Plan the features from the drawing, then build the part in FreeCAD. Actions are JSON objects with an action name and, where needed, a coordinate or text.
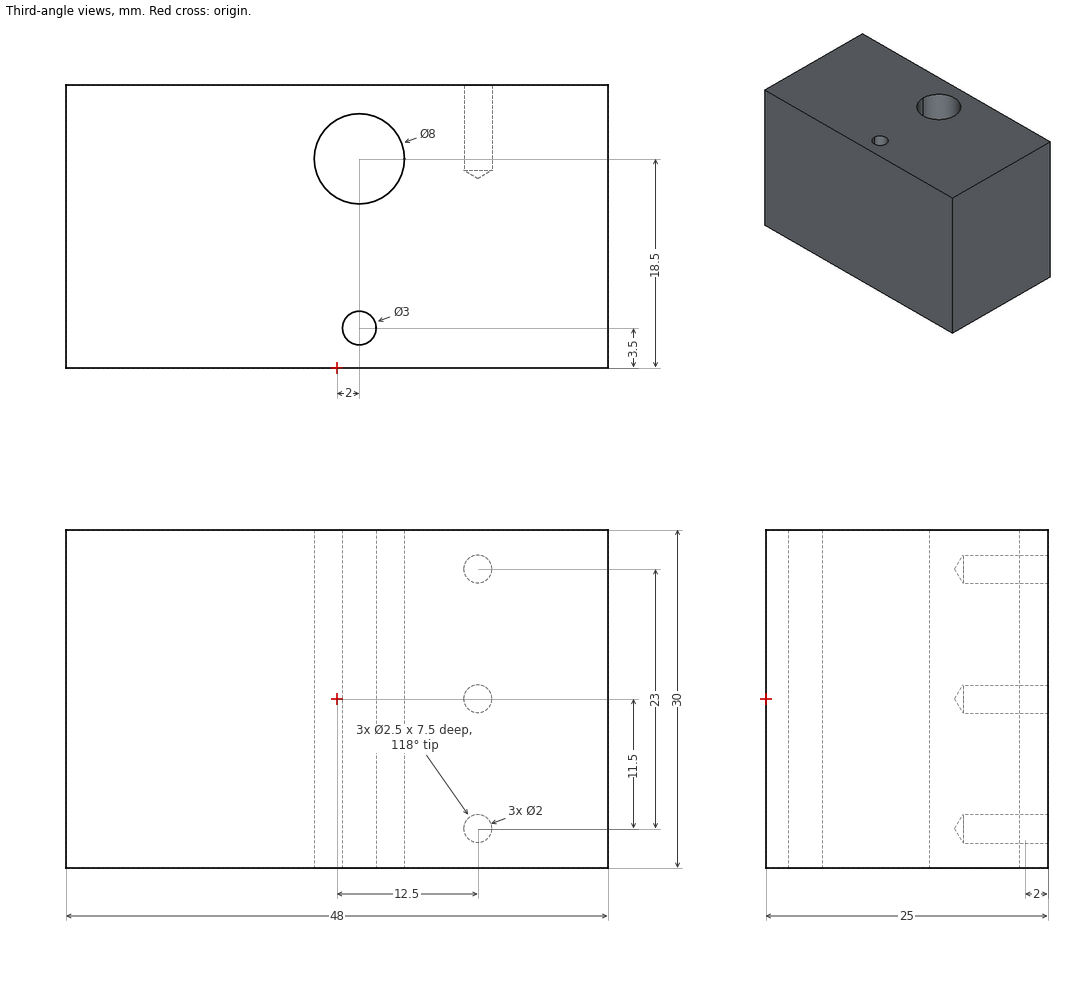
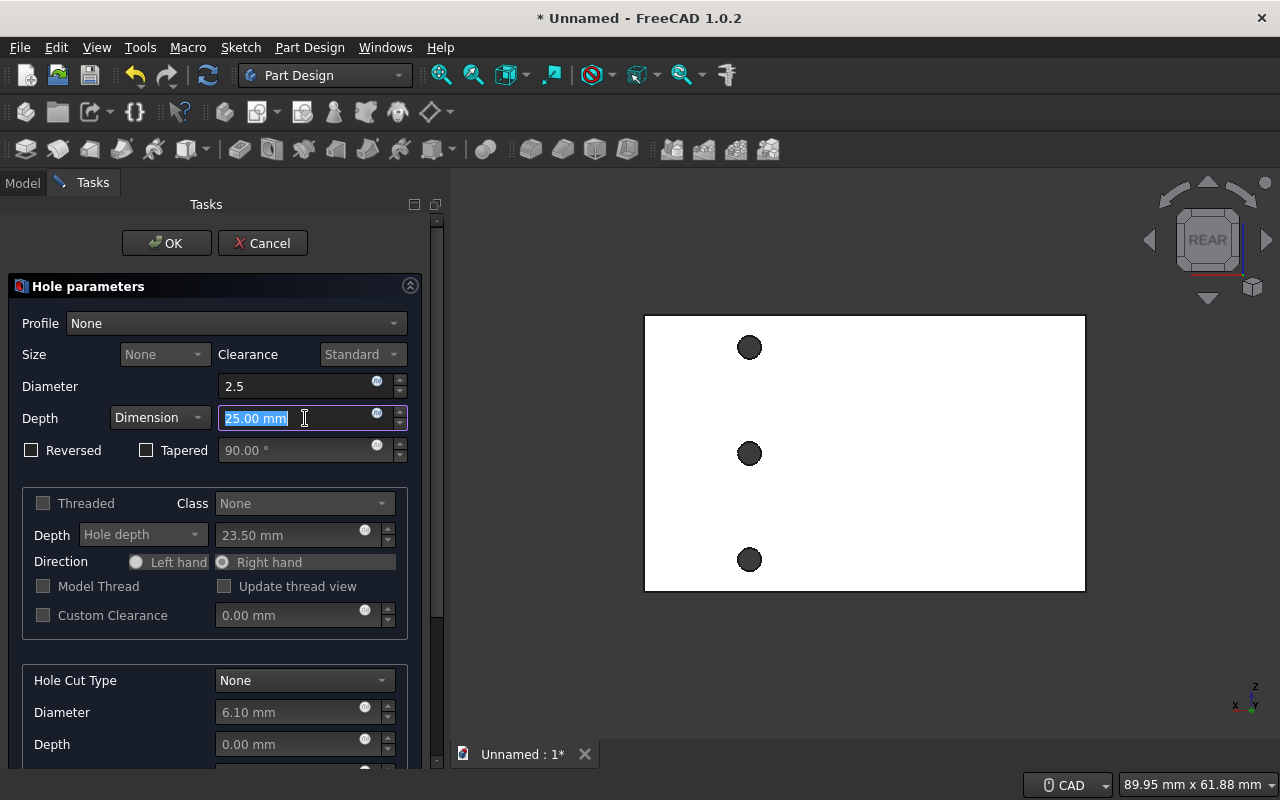
{"action": "type", "text": "7.5"}
{"action": "key", "text": "Tab"}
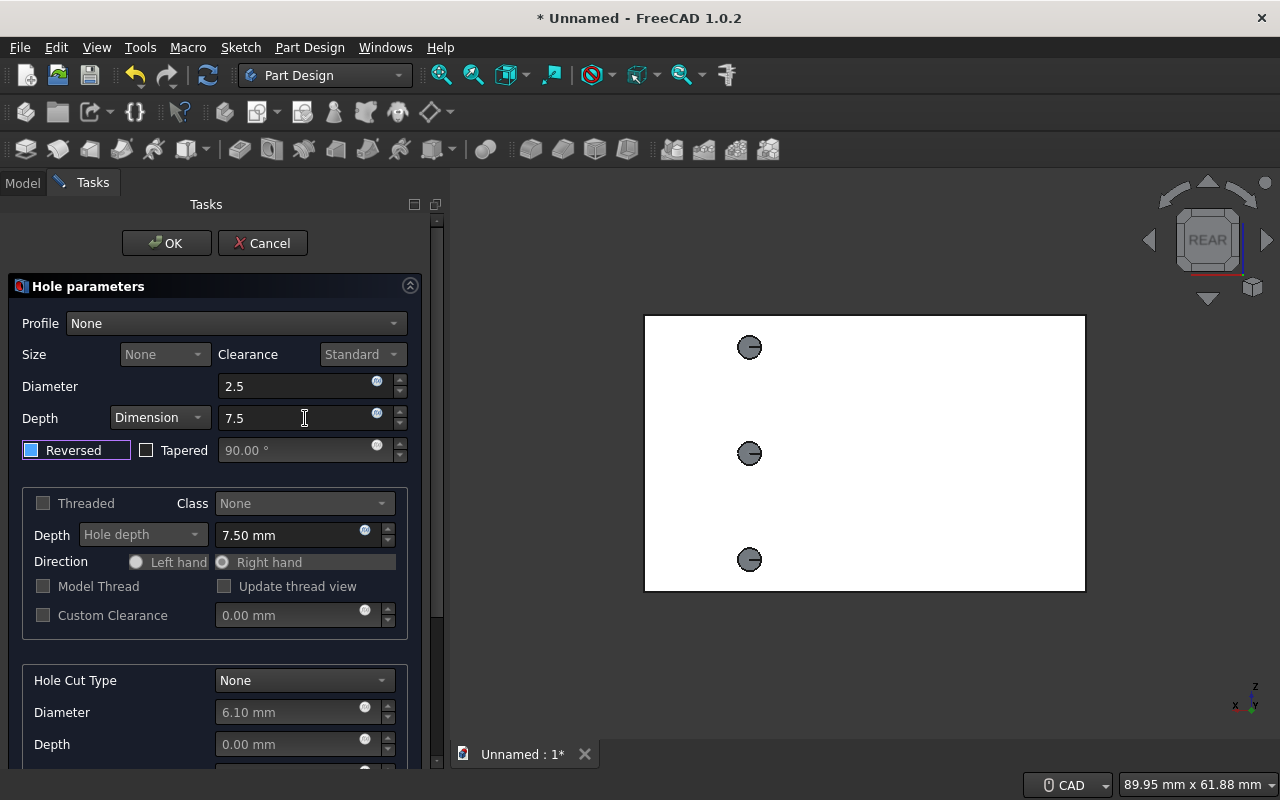
{"action": "left_click", "coordinate": [167, 243]}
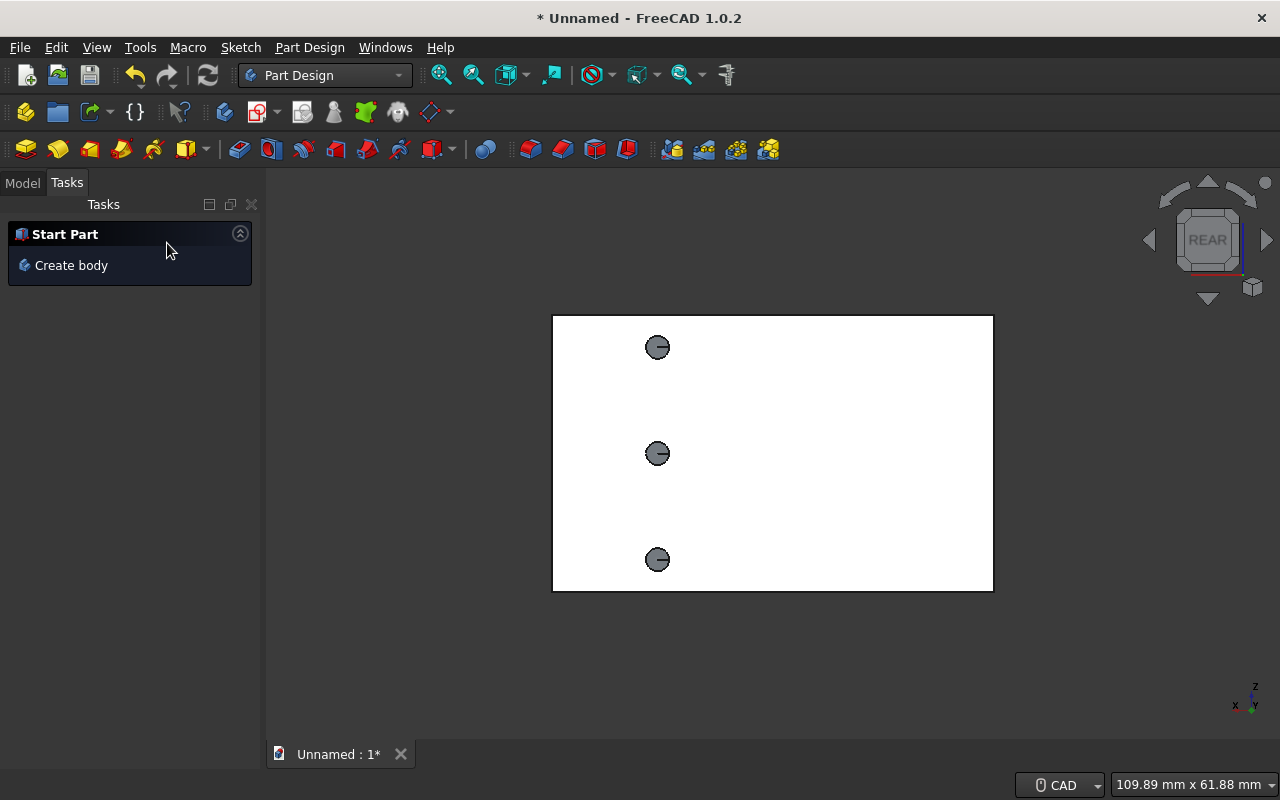
{"action": "key", "text": "0"}